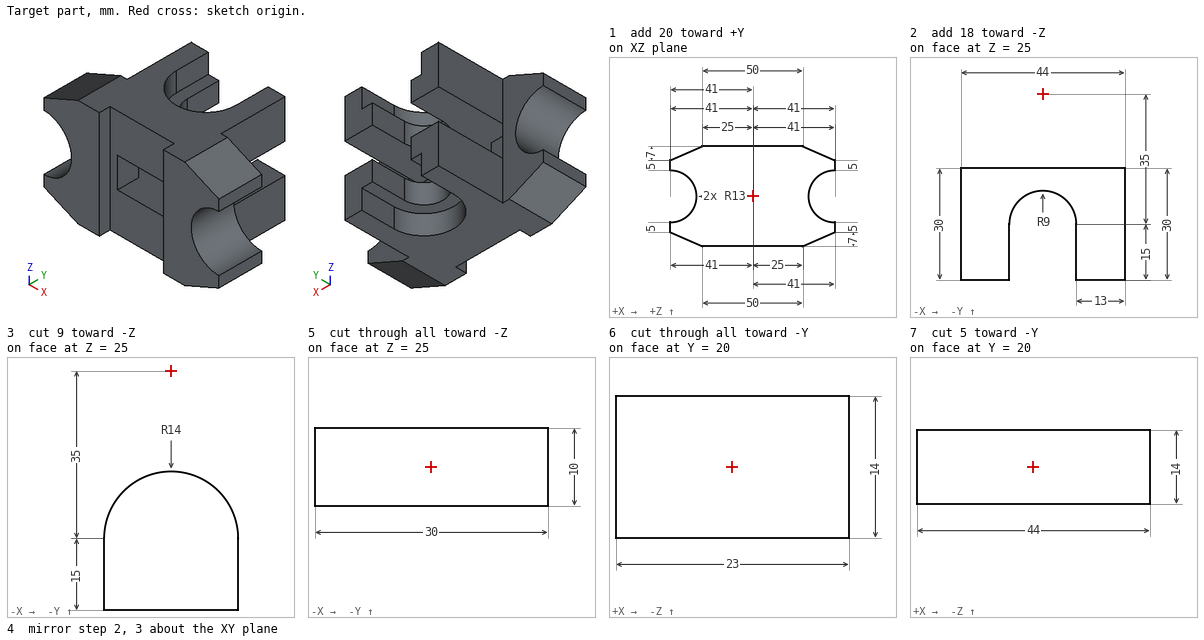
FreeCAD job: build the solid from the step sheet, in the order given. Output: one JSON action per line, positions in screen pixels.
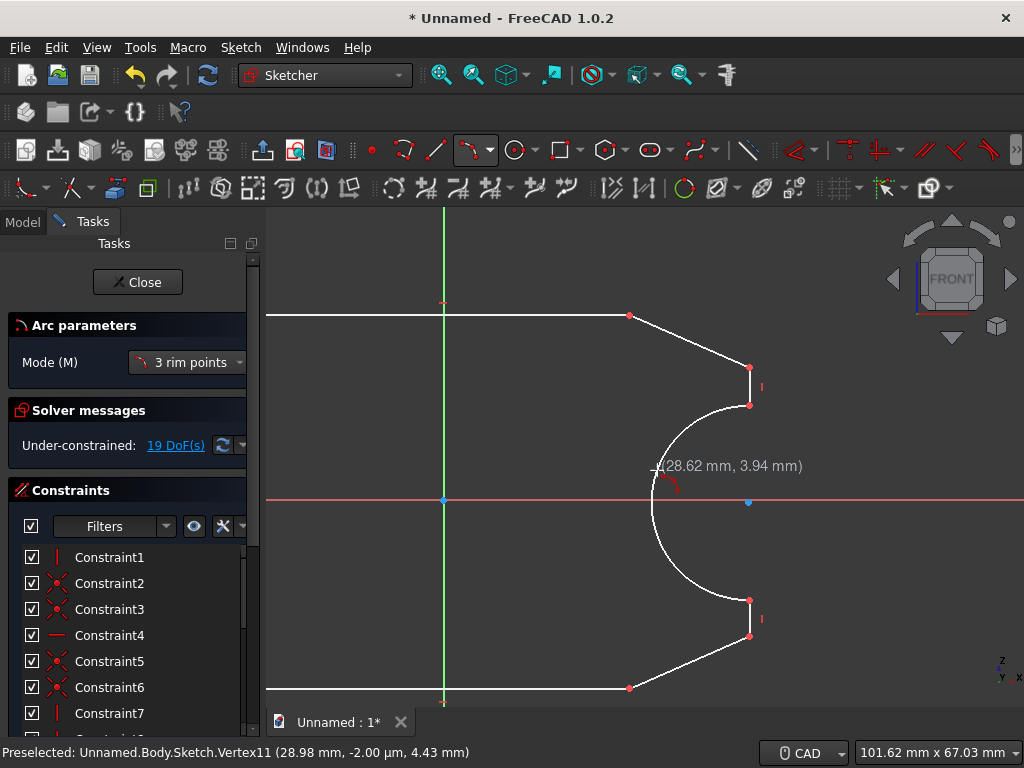
{"action": "scroll", "coordinate": [847, 369], "scroll_direction": "down", "scroll_amount": 2}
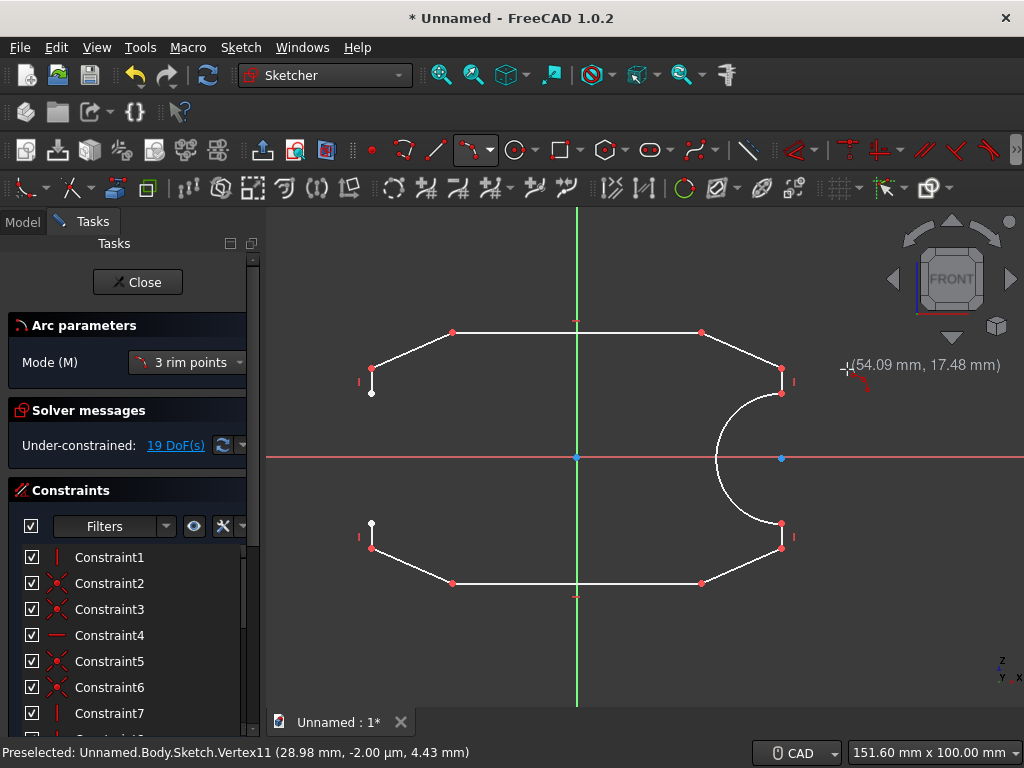
{"action": "scroll", "coordinate": [372, 522], "scroll_direction": "up", "scroll_amount": 2}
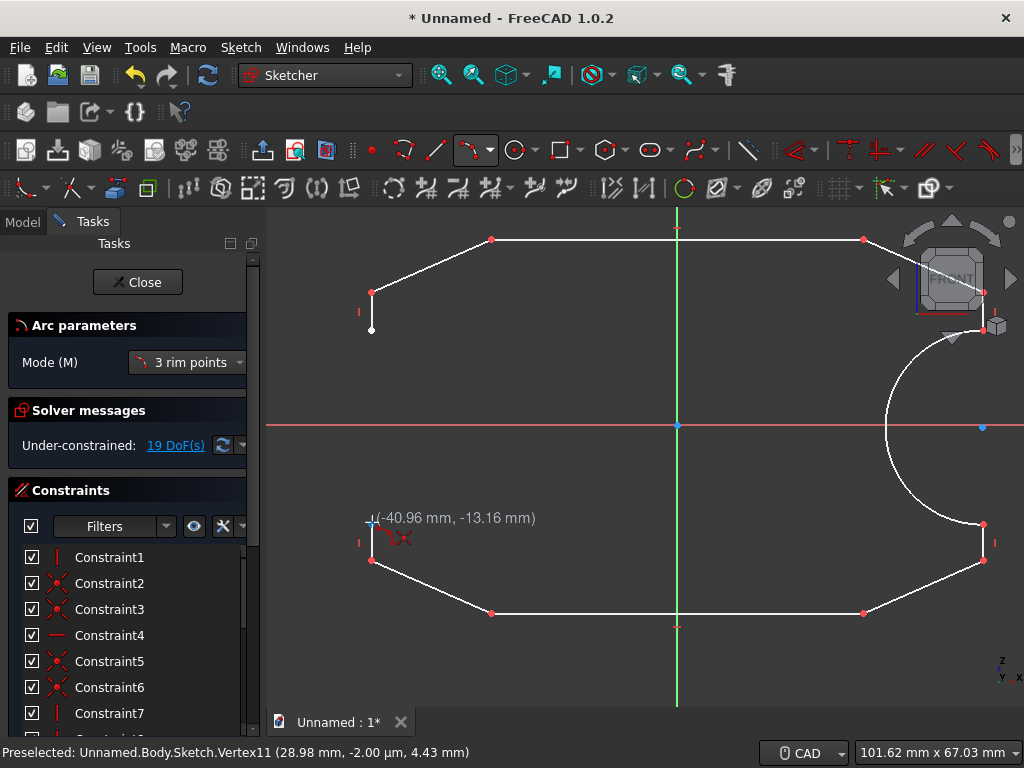
{"action": "left_click", "coordinate": [372, 525]}
{"action": "left_click", "coordinate": [372, 330]}
{"action": "left_click", "coordinate": [464, 455]}
{"action": "key", "text": "Escape"}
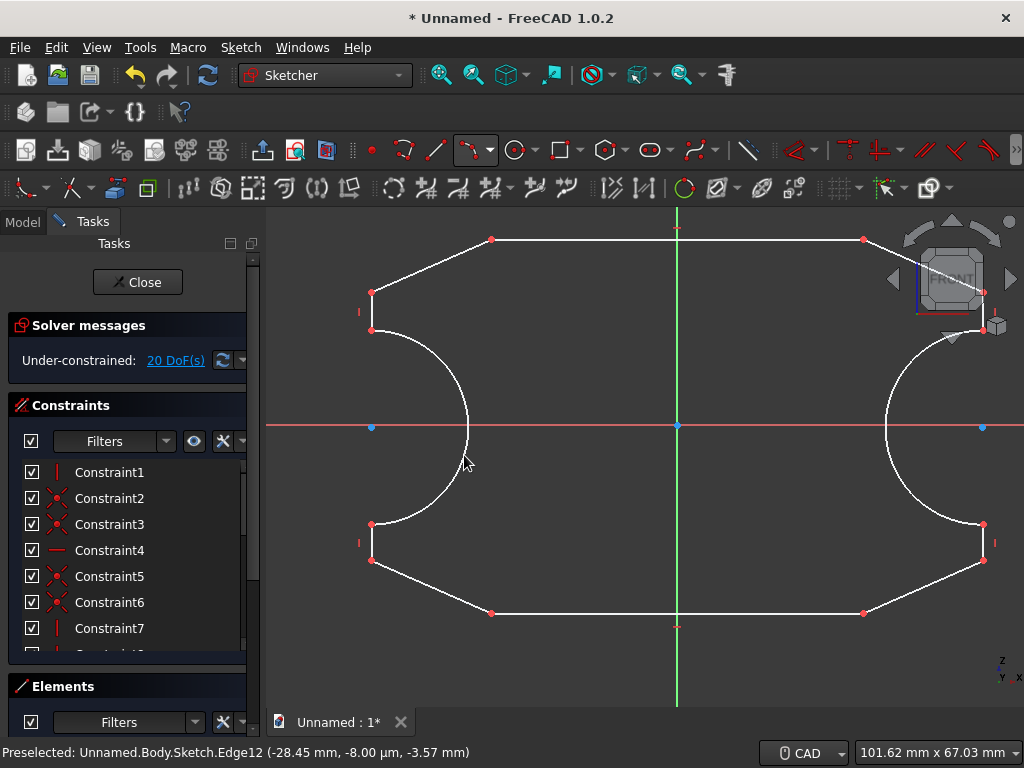
{"action": "scroll", "coordinate": [371, 522], "scroll_direction": "down", "scroll_amount": 2}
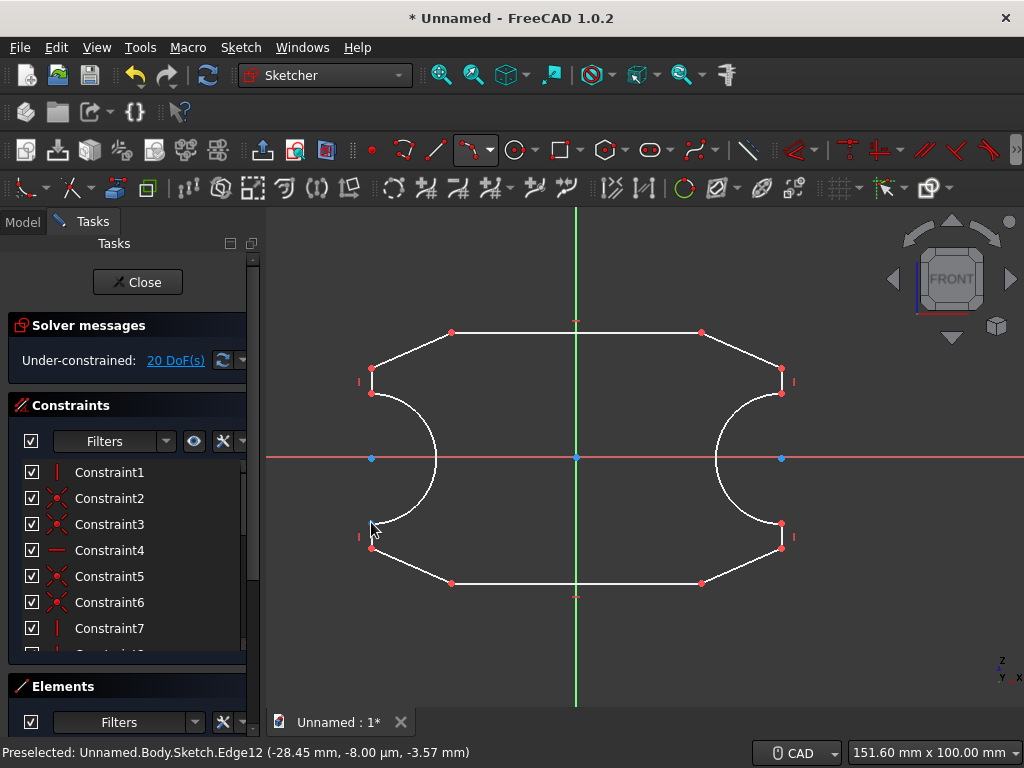
{"action": "left_click", "coordinate": [728, 420]}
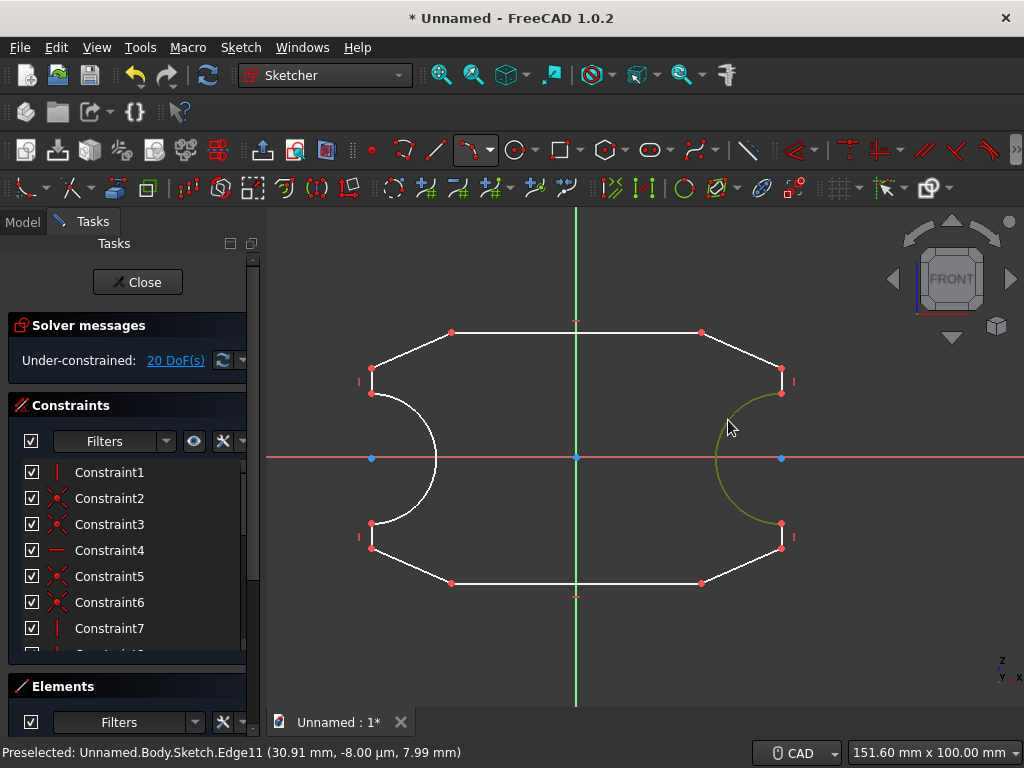
{"action": "left_click", "coordinate": [424, 497]}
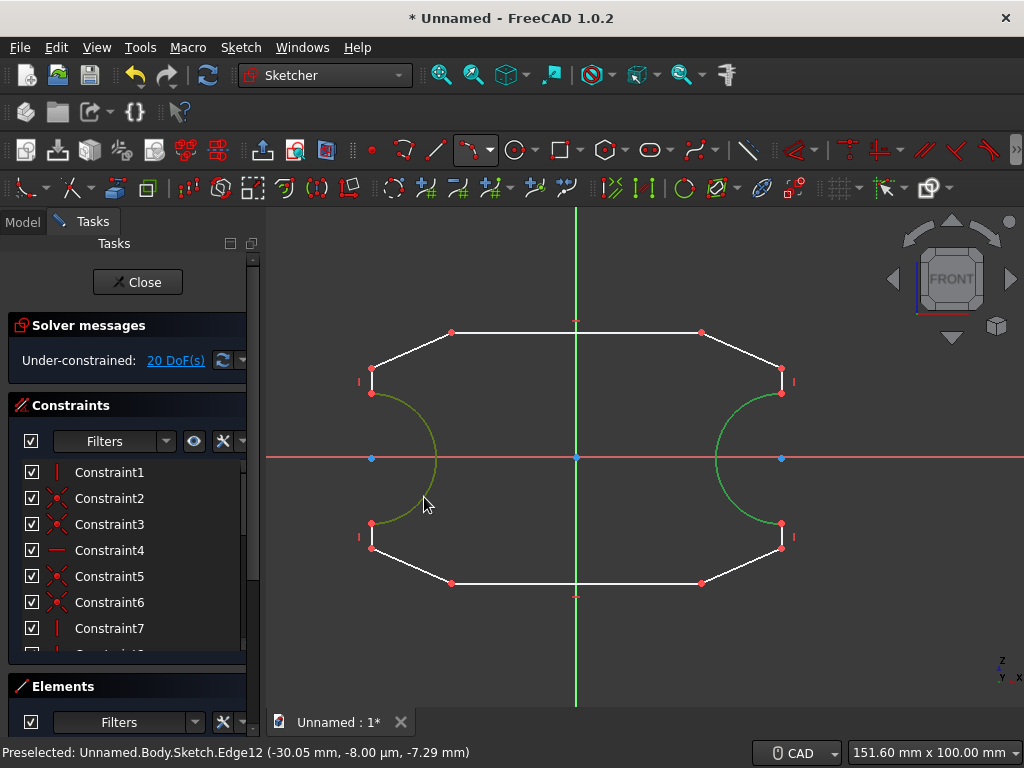
{"action": "key", "text": "e"}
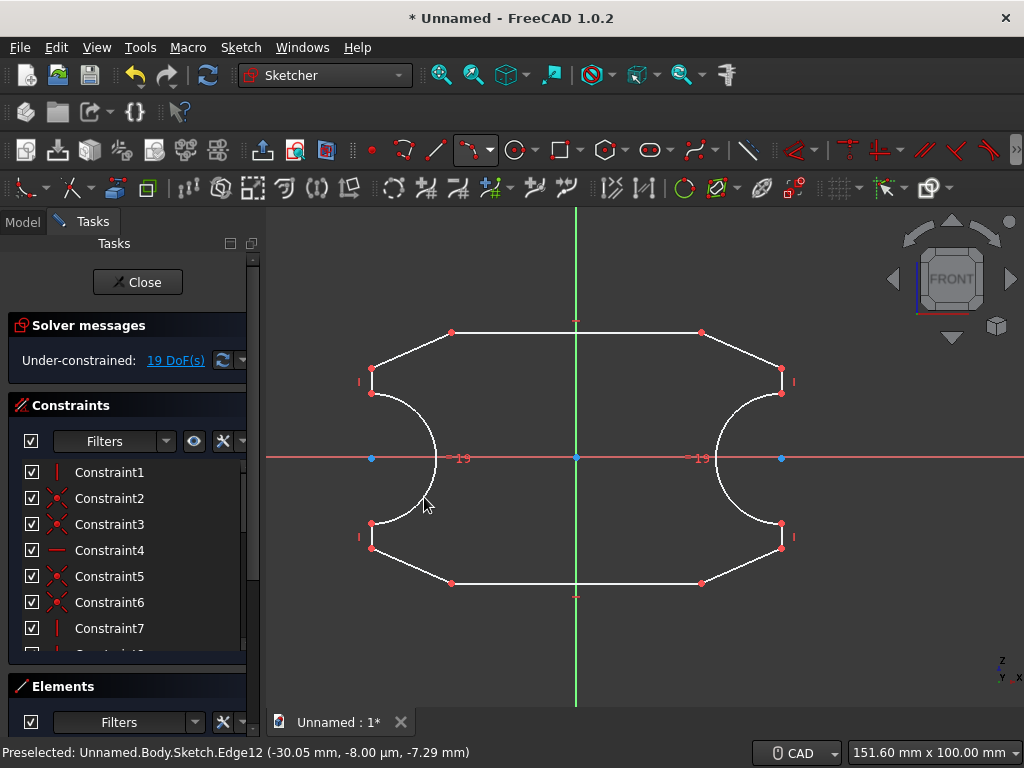
{"action": "left_click", "coordinate": [781, 459]}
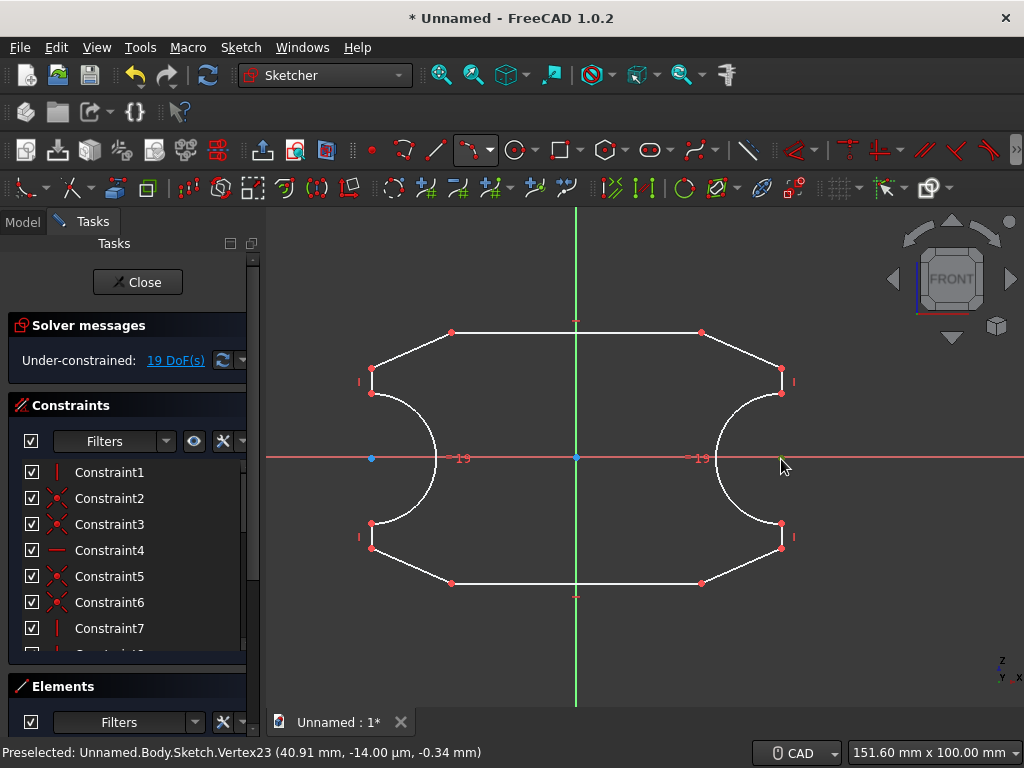
{"action": "left_click", "coordinate": [334, 457]}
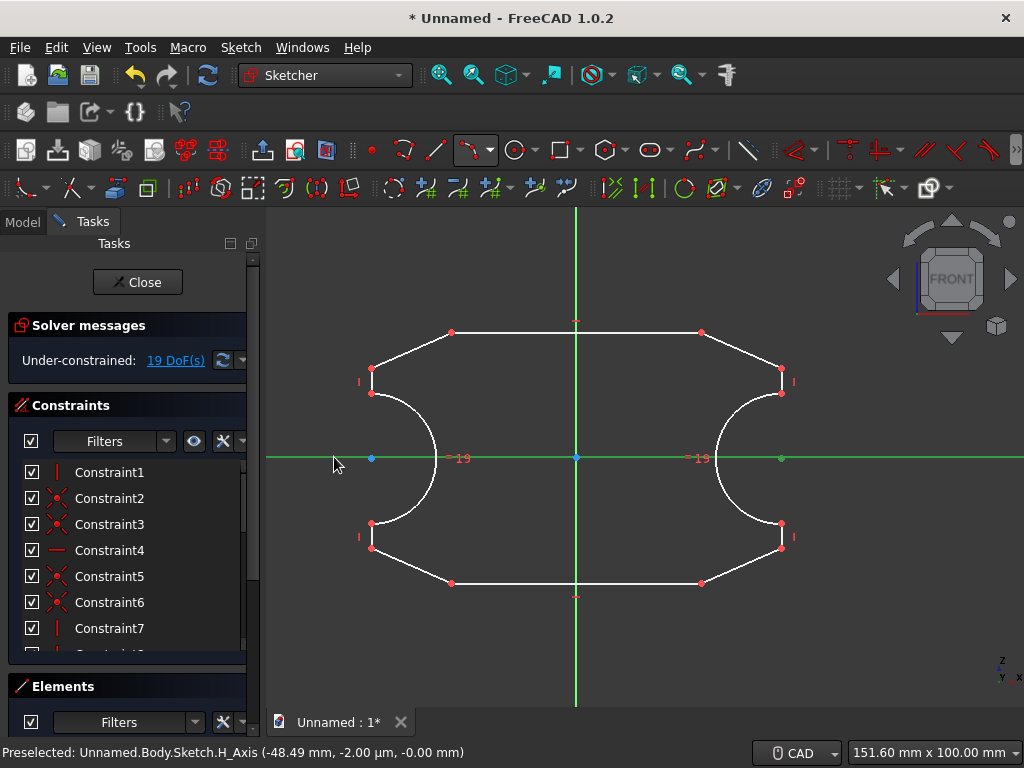
{"action": "left_click", "coordinate": [848, 150]}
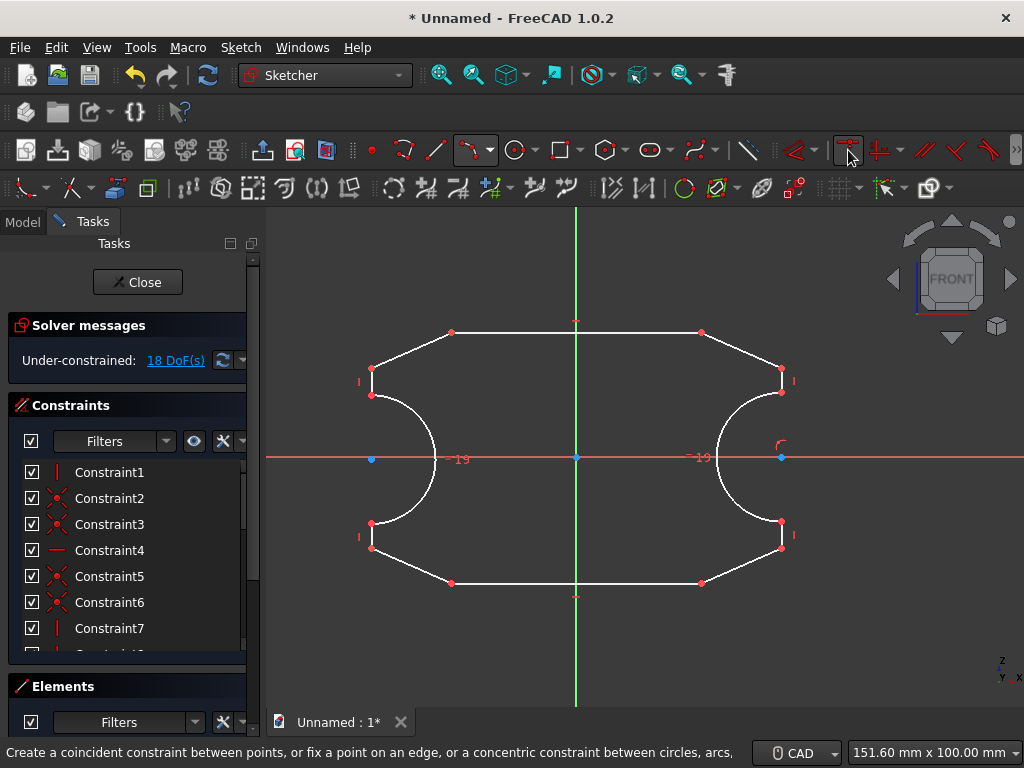
{"action": "left_click", "coordinate": [371, 460]}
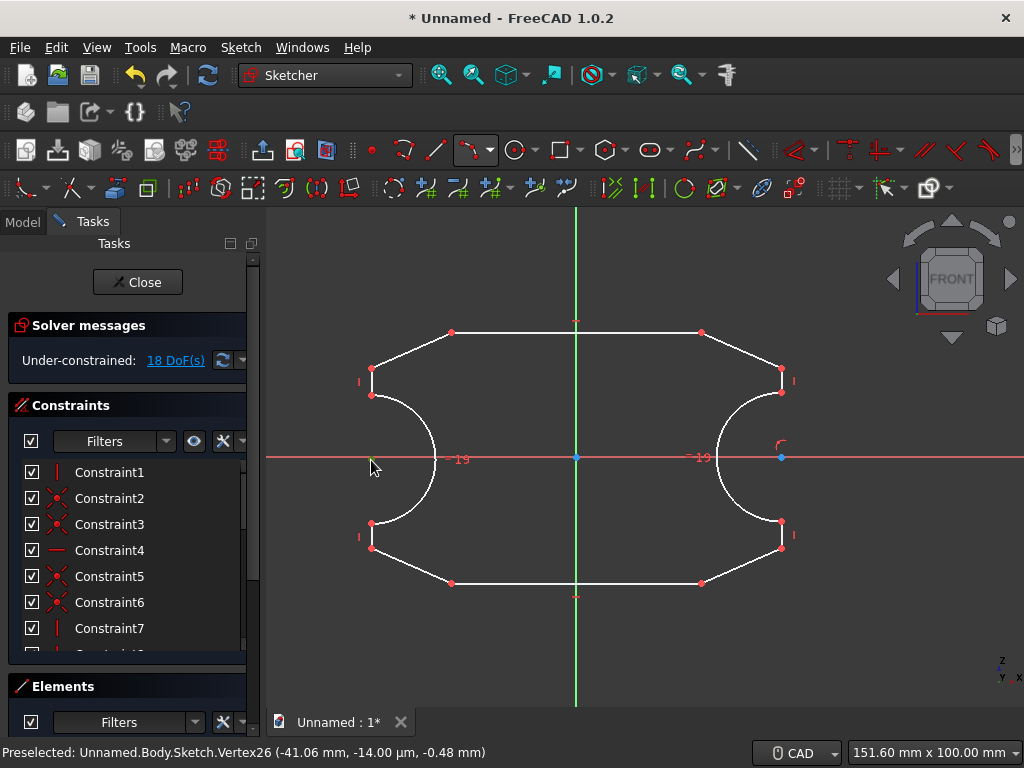
{"action": "left_click", "coordinate": [334, 457]}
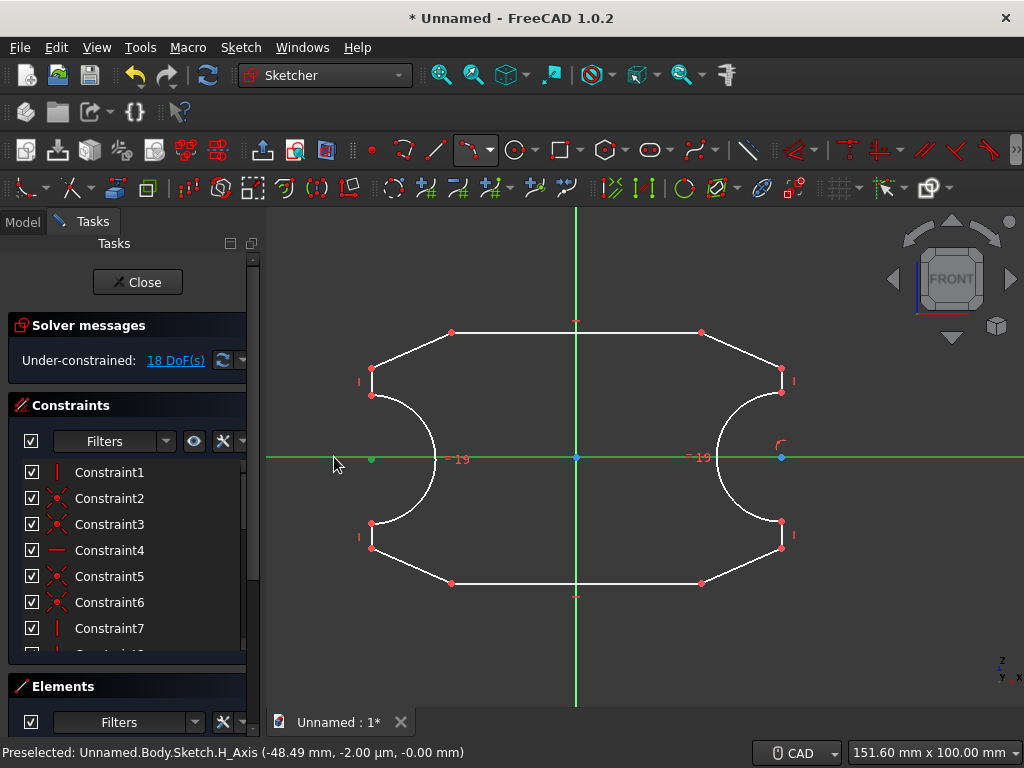
{"action": "left_click", "coordinate": [848, 150]}